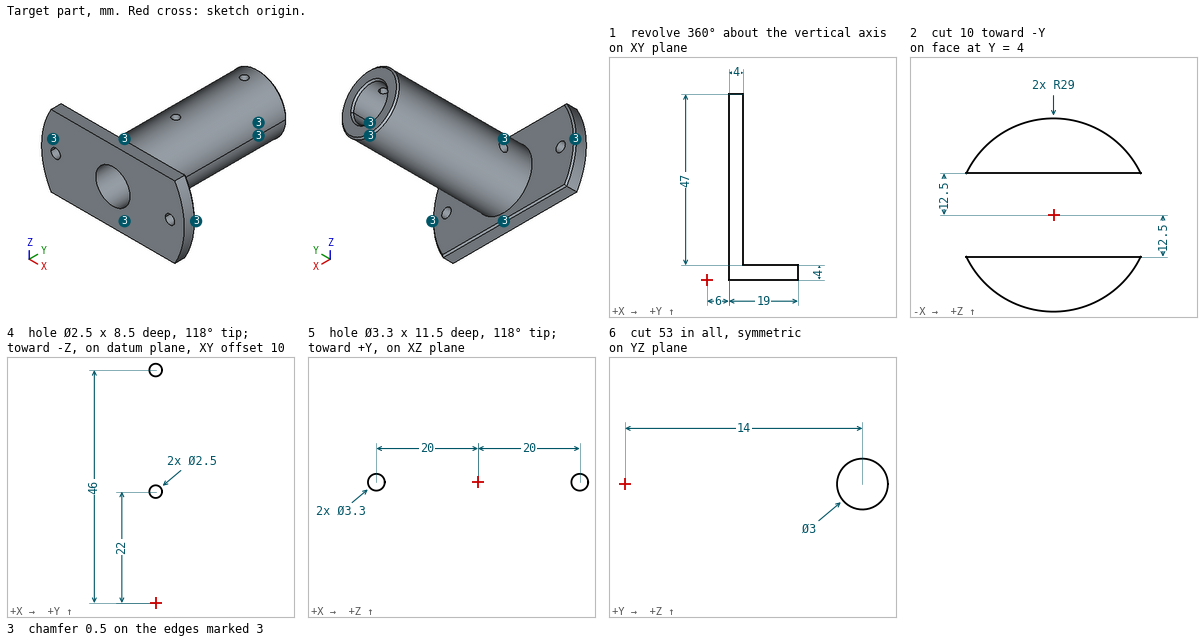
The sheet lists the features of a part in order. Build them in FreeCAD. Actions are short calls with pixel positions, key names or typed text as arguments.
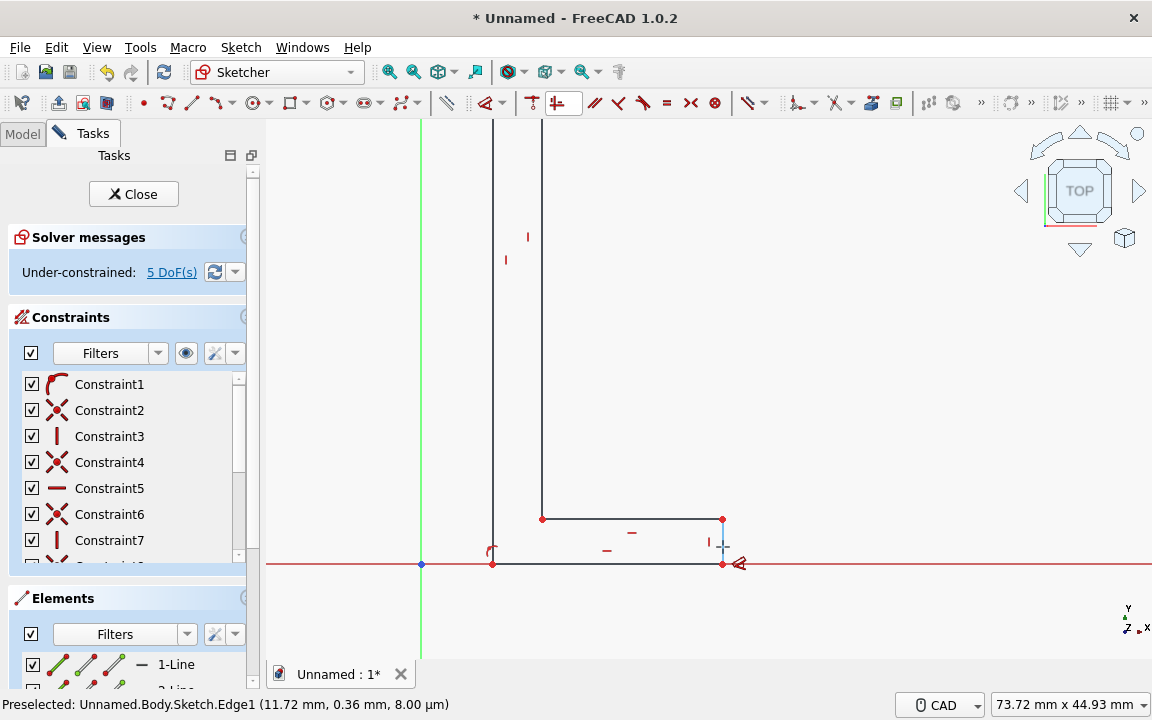
click(723, 546)
click(757, 542)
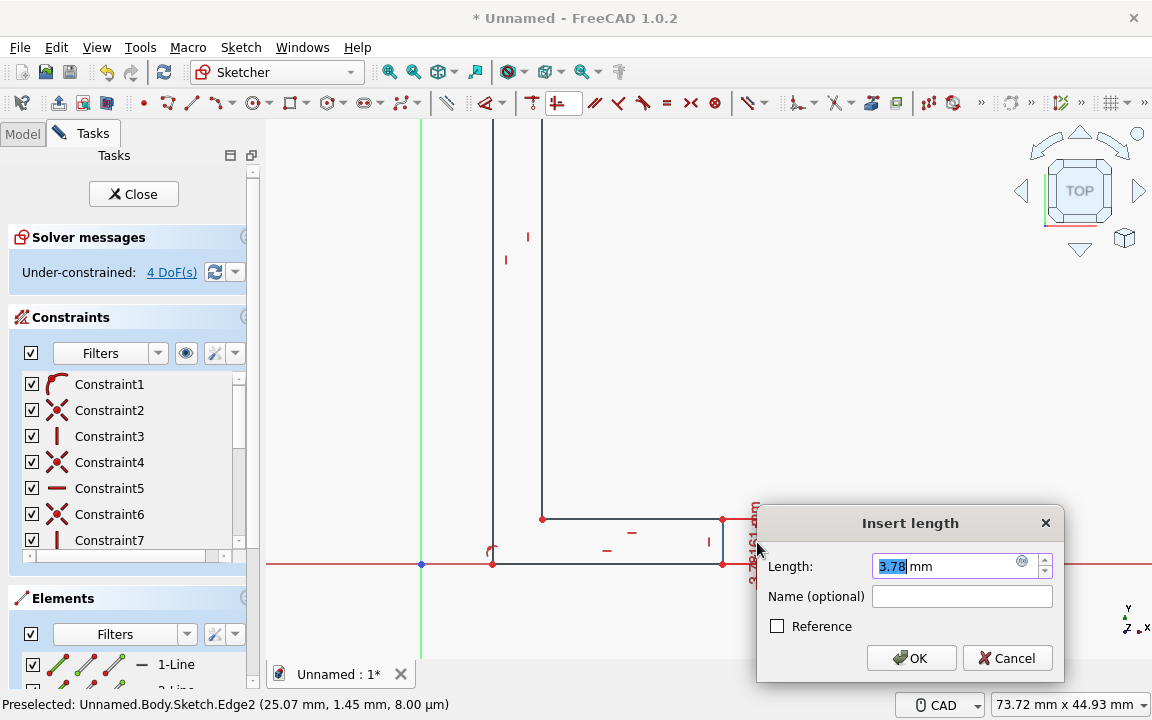
text(4)
key(Return)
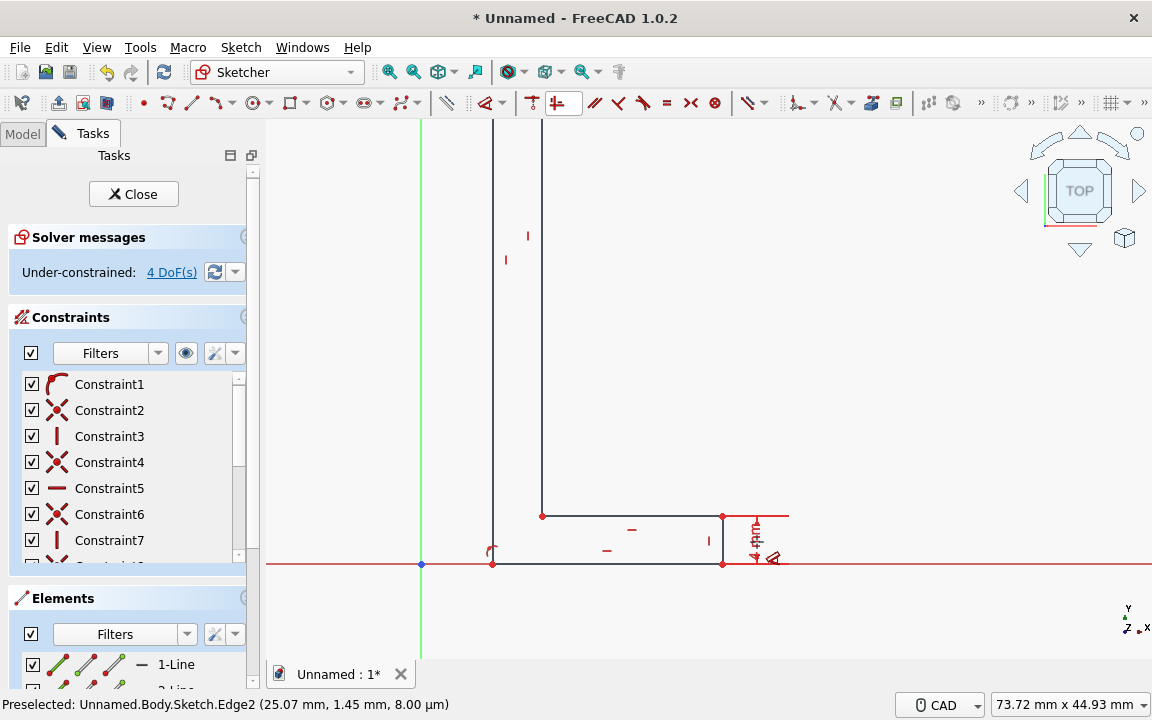
scroll(724, 548, down, 3)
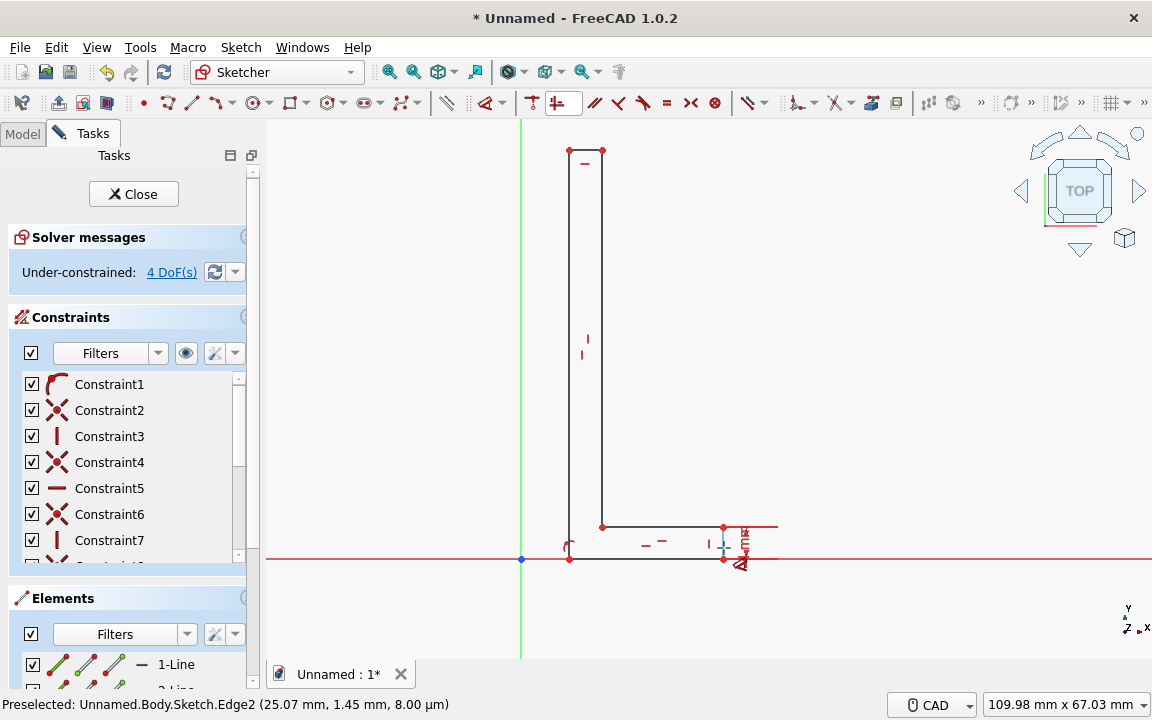
scroll(616, 222, up, 3)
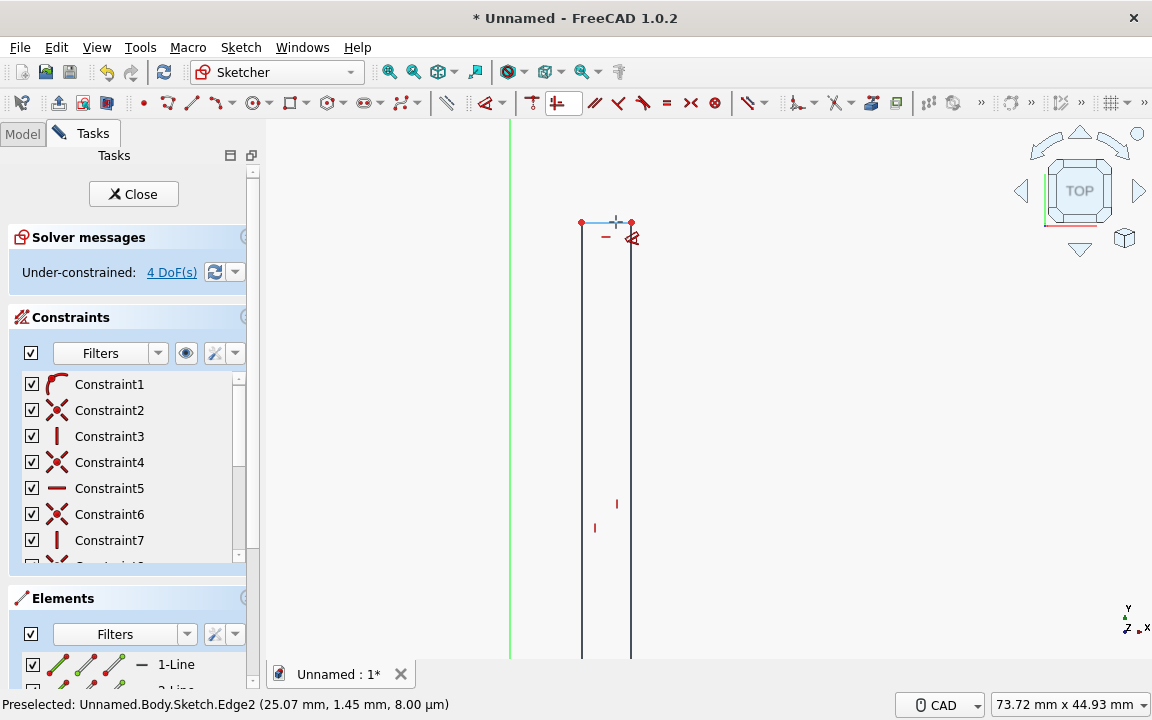
click(616, 223)
click(606, 189)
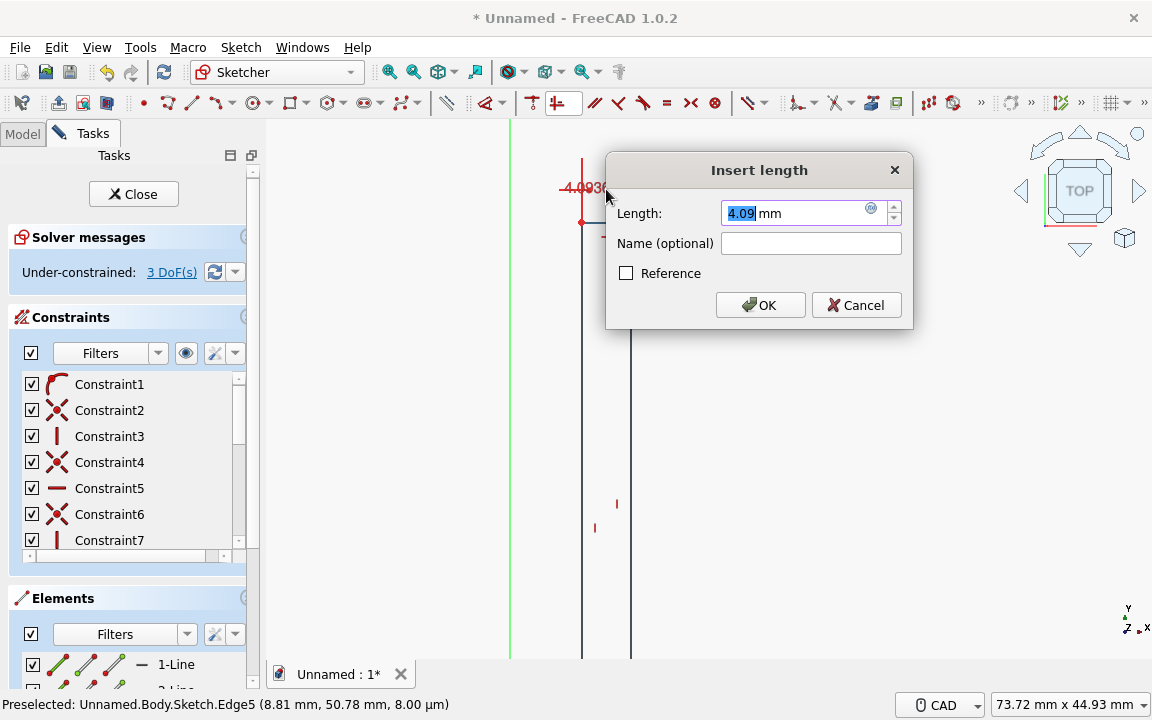
text(4)
key(Return)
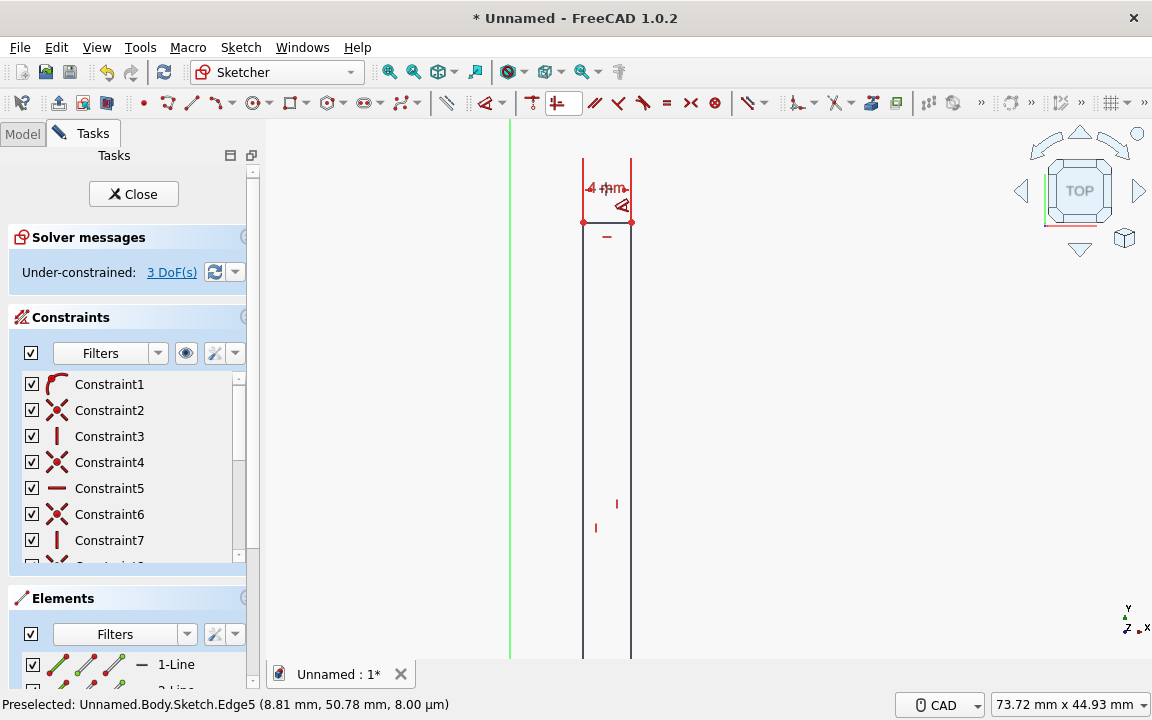
scroll(616, 222, down, 3)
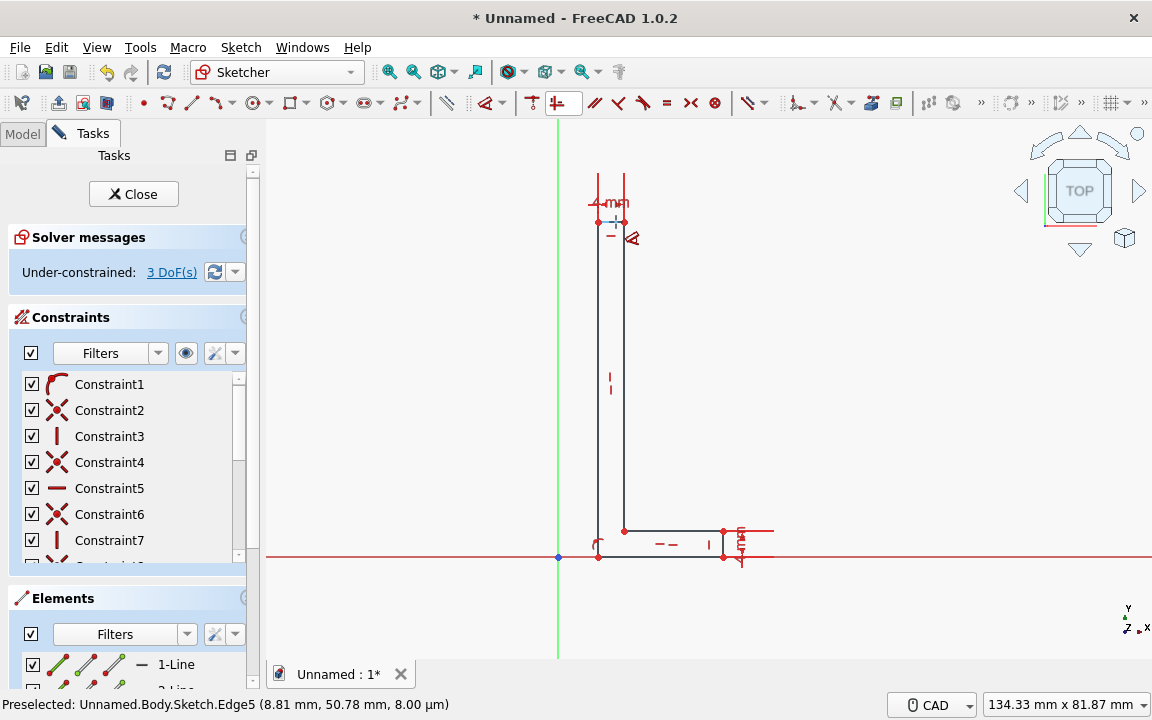
click(636, 557)
click(661, 591)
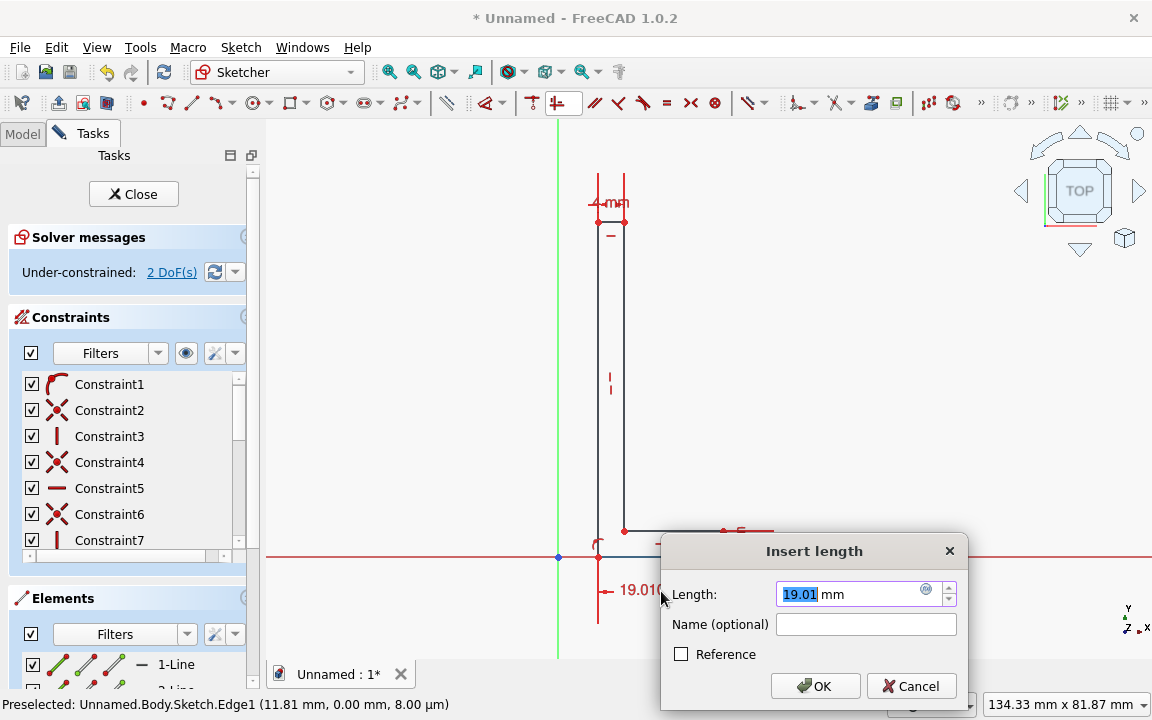
text(19)
key(Return)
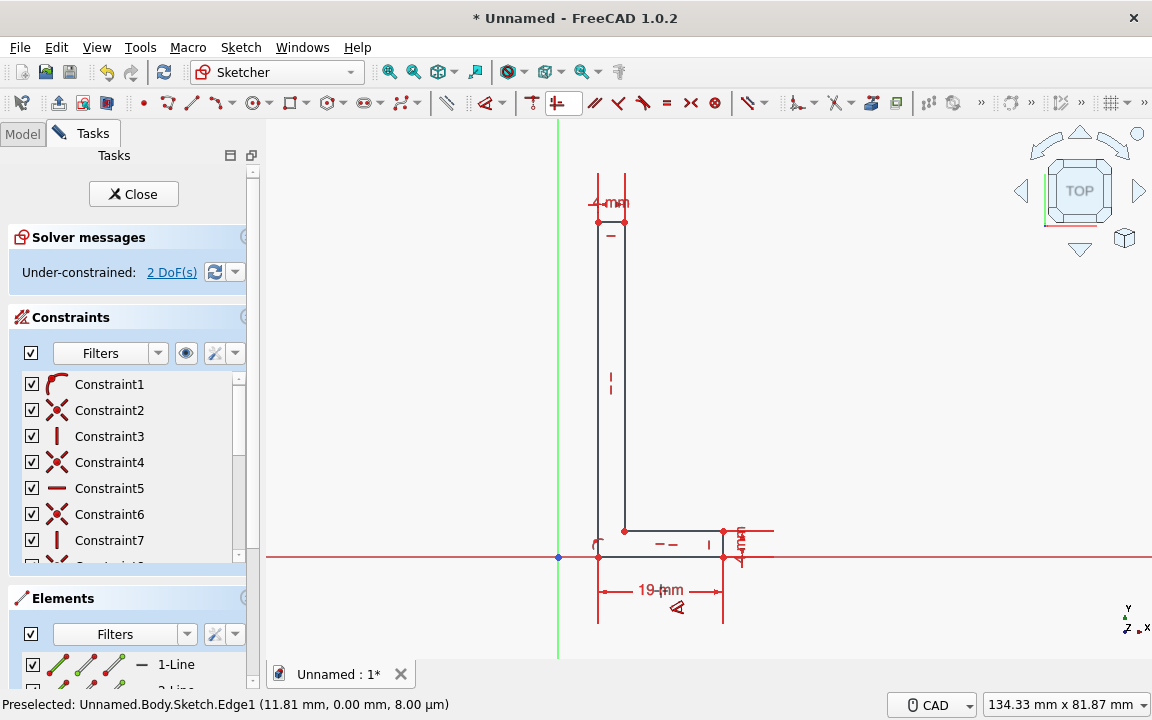
click(625, 438)
click(659, 377)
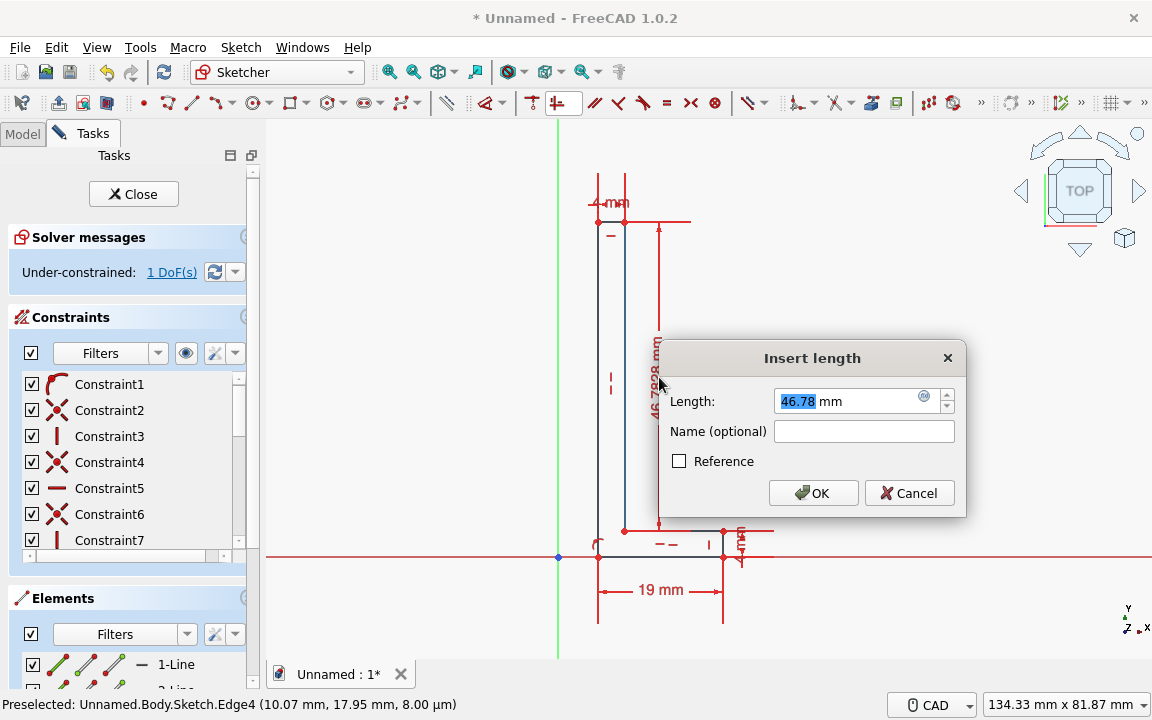
text(47)
key(Return)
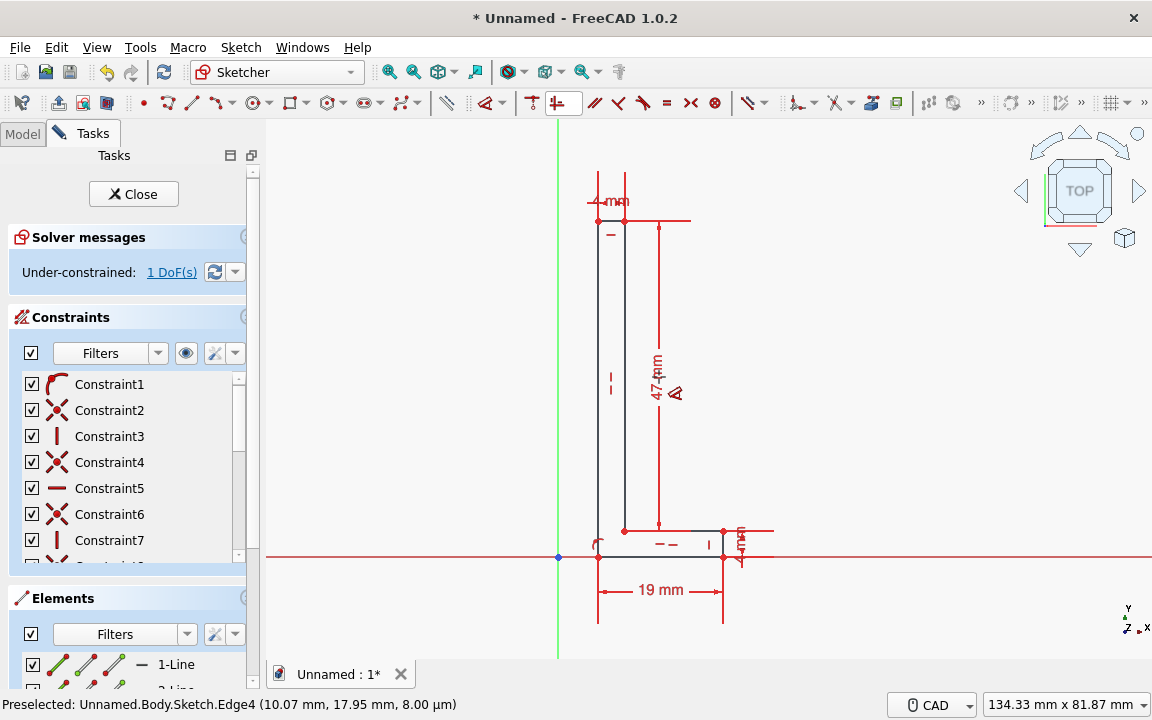
click(598, 557)
click(578, 591)